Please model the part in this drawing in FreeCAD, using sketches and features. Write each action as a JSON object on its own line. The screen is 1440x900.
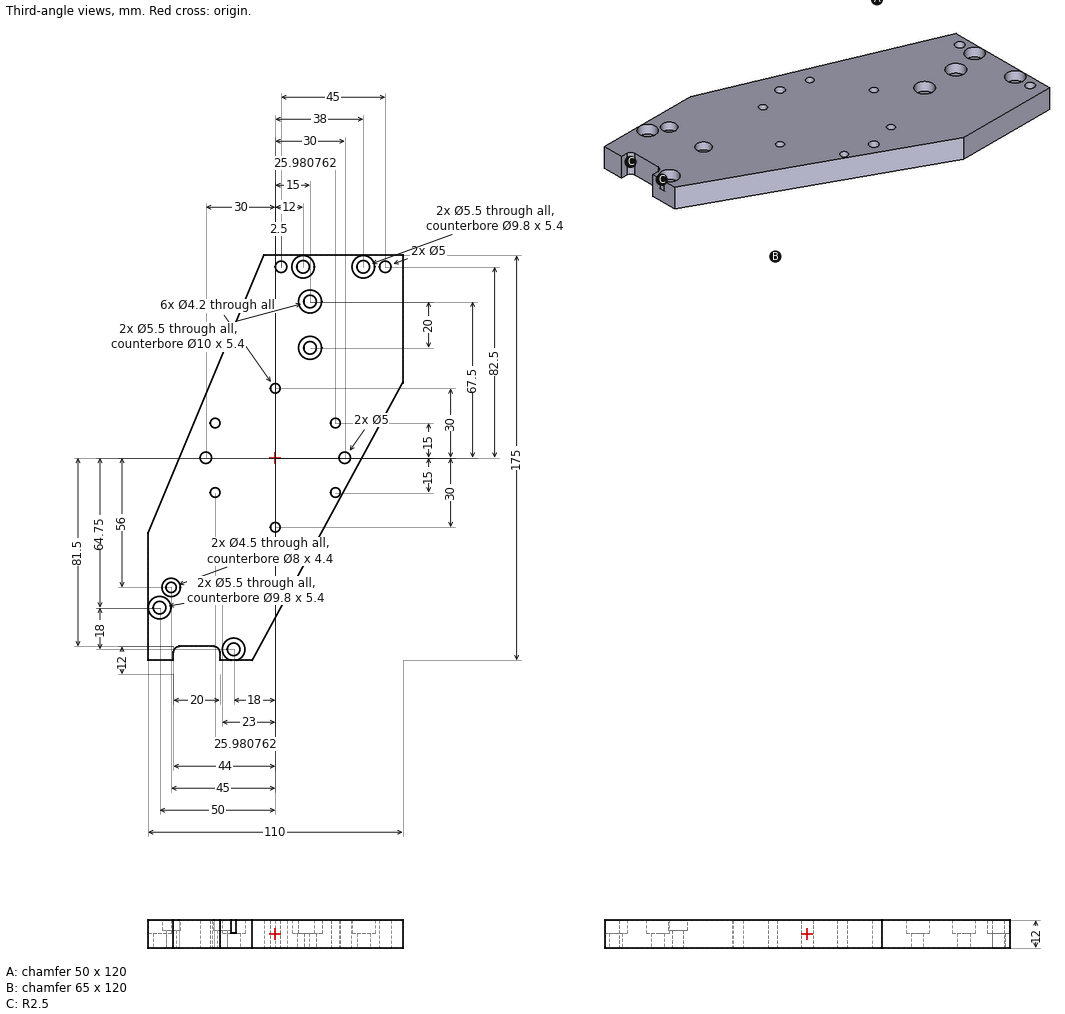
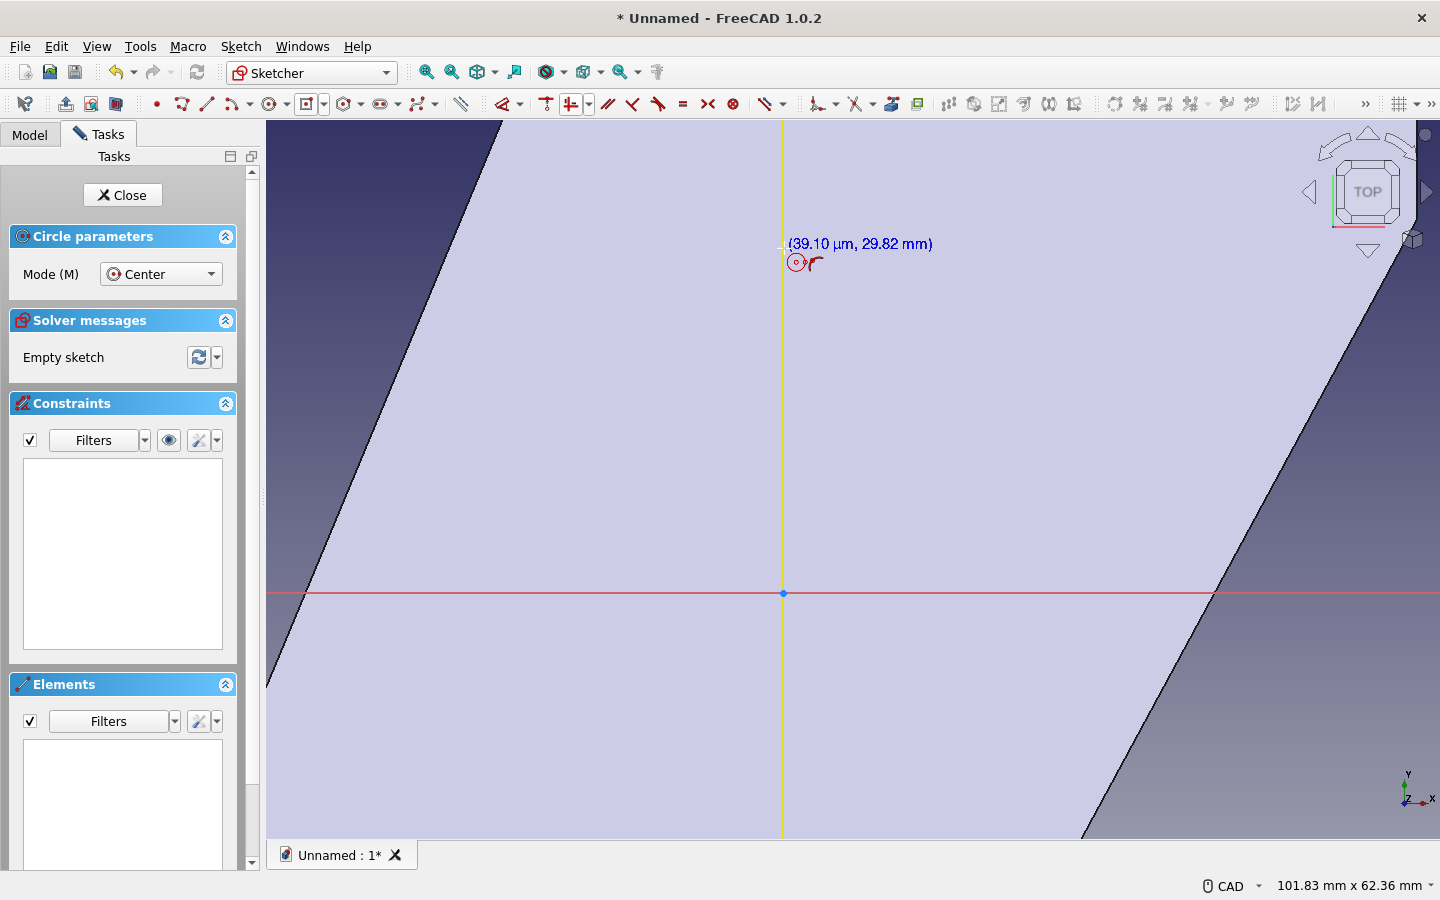
{"action": "left_click", "coordinate": [783, 247]}
{"action": "left_click", "coordinate": [800, 230]}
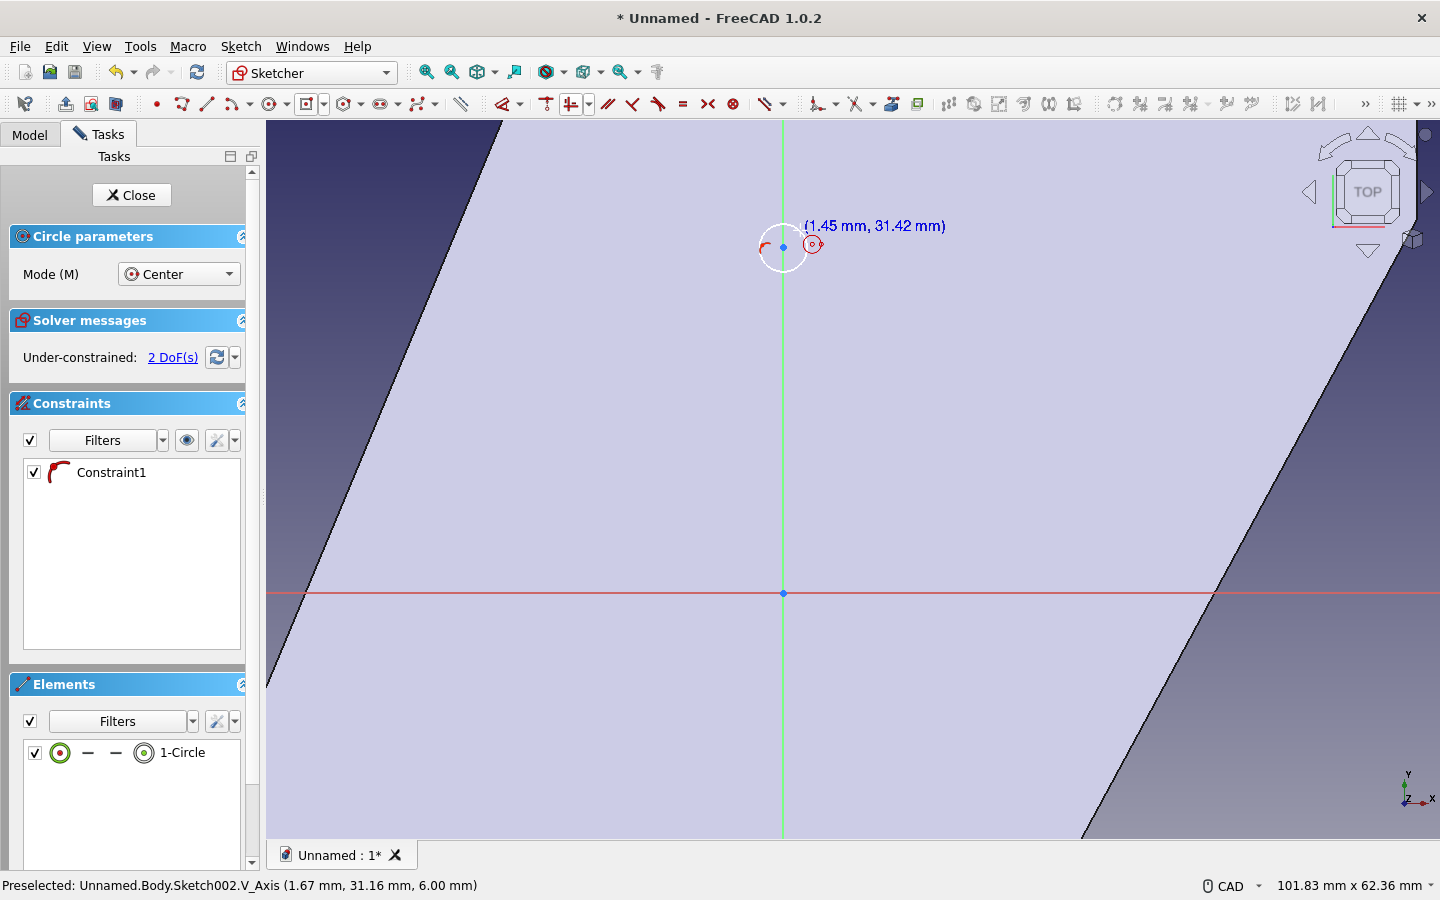
{"action": "left_click", "coordinate": [1083, 420]}
{"action": "left_click", "coordinate": [1100, 403]}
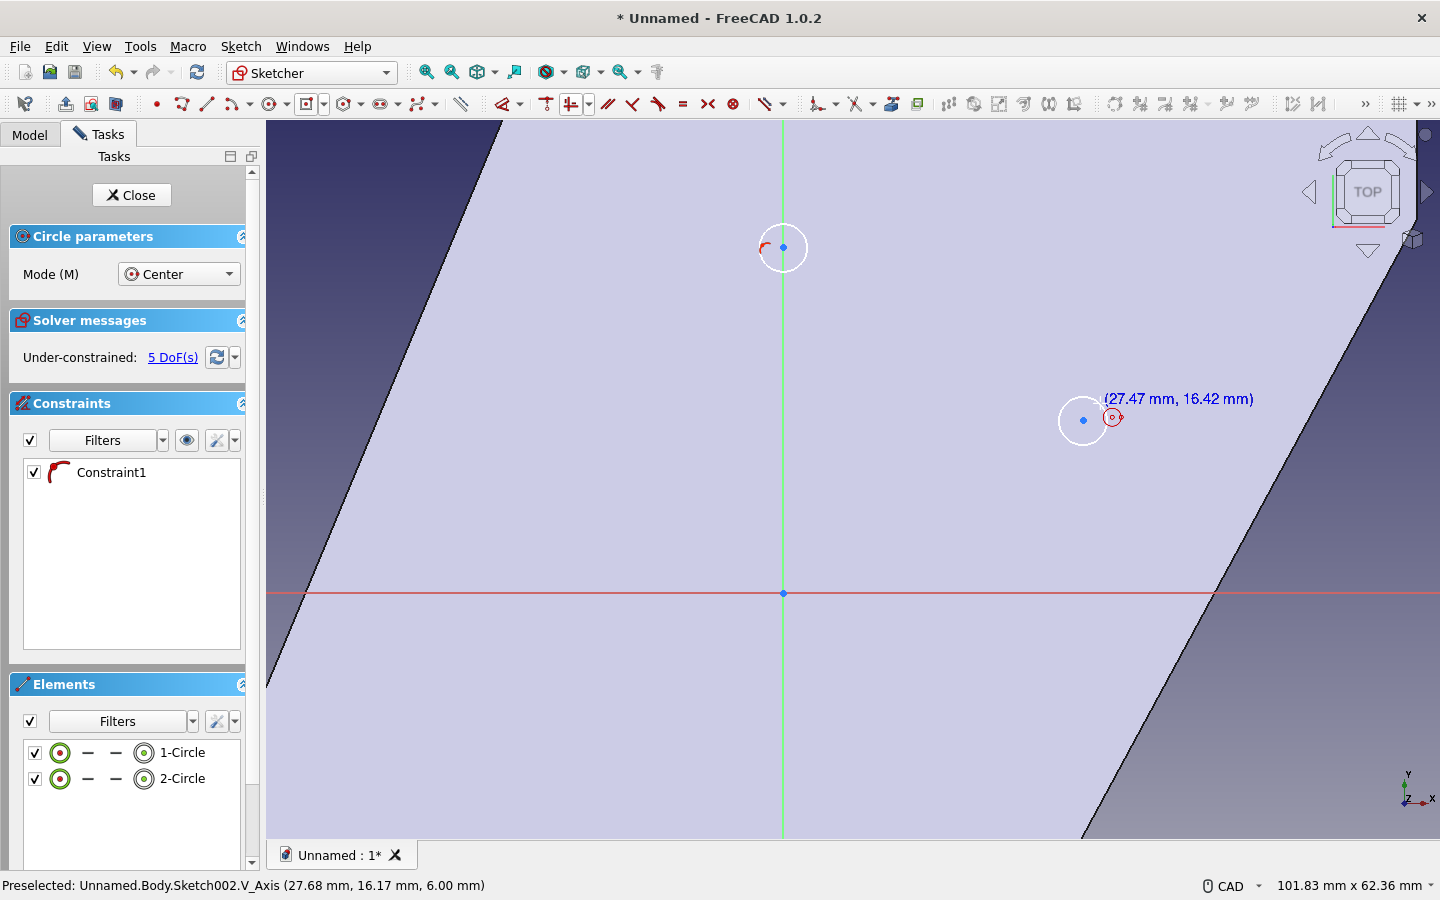
{"action": "left_click", "coordinate": [1083, 766]}
{"action": "left_click", "coordinate": [1100, 749]}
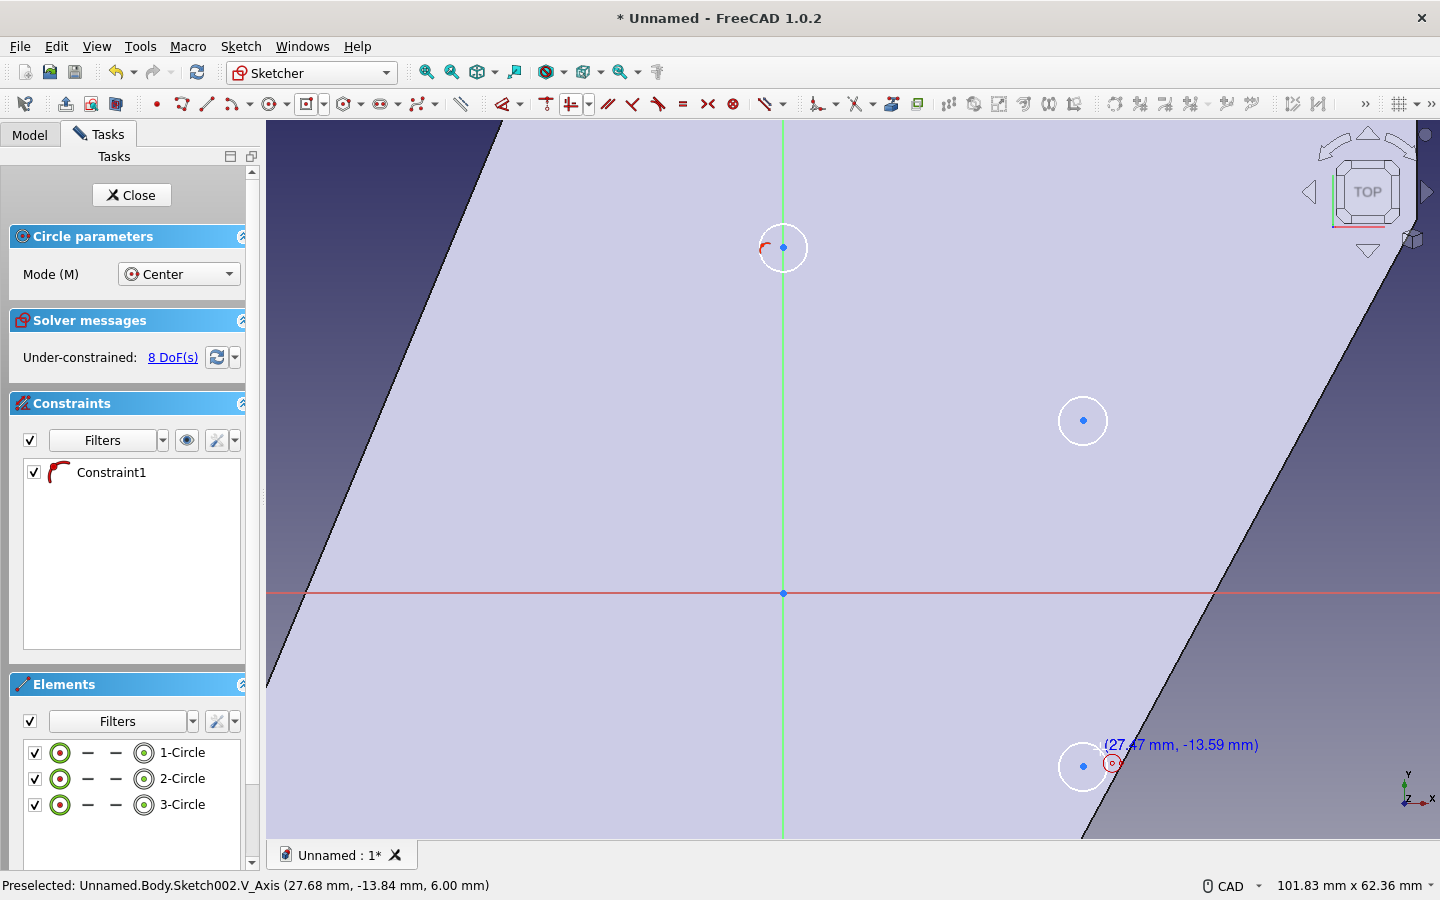
{"action": "scroll", "coordinate": [787, 248], "scroll_direction": "down", "scroll_amount": 2}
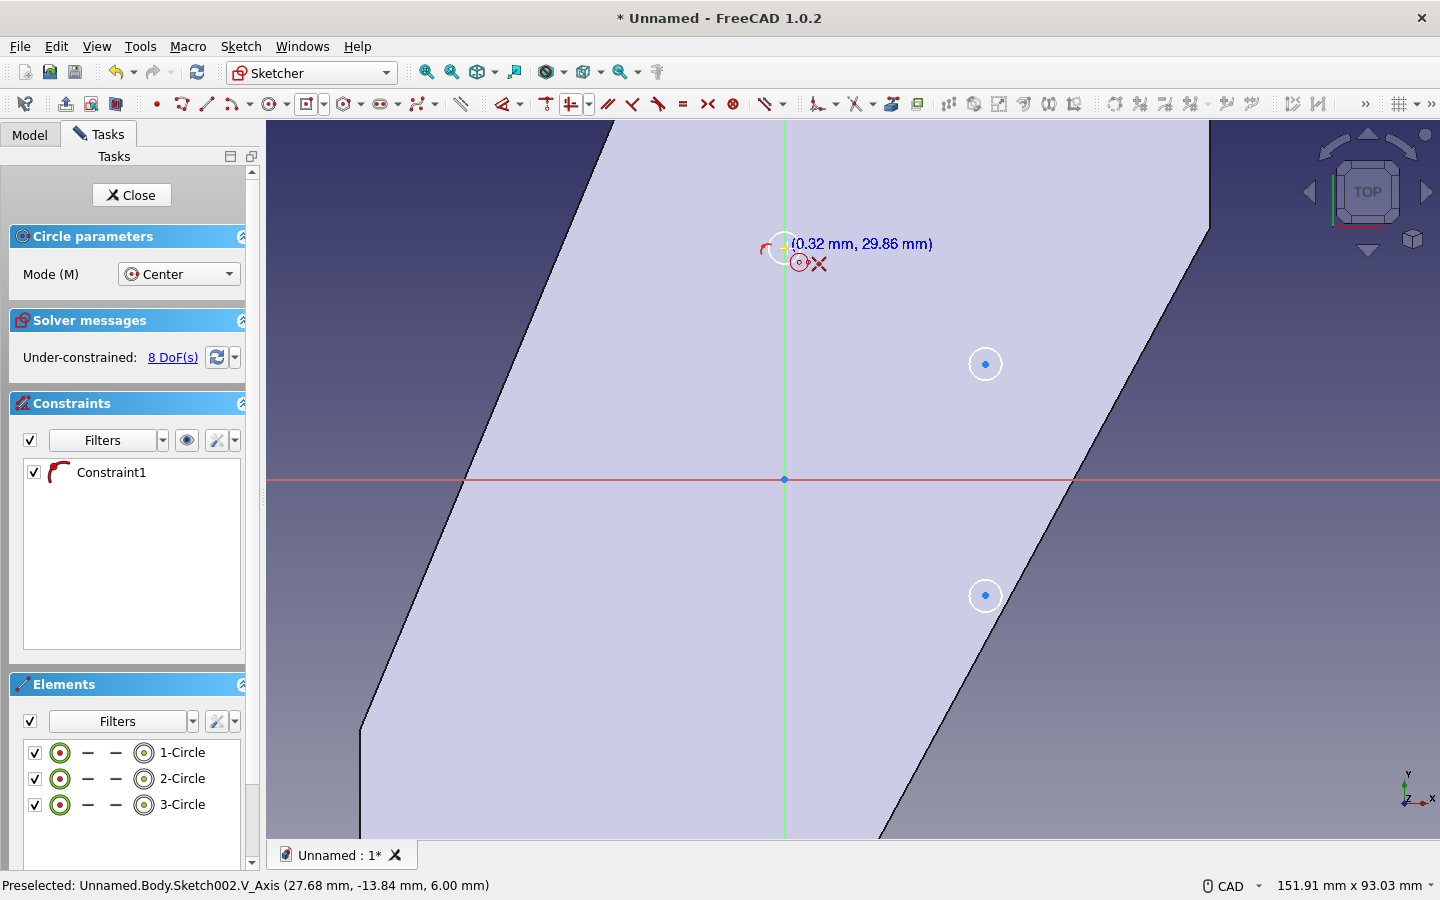
{"action": "scroll", "coordinate": [785, 711], "scroll_direction": "up", "scroll_amount": 2}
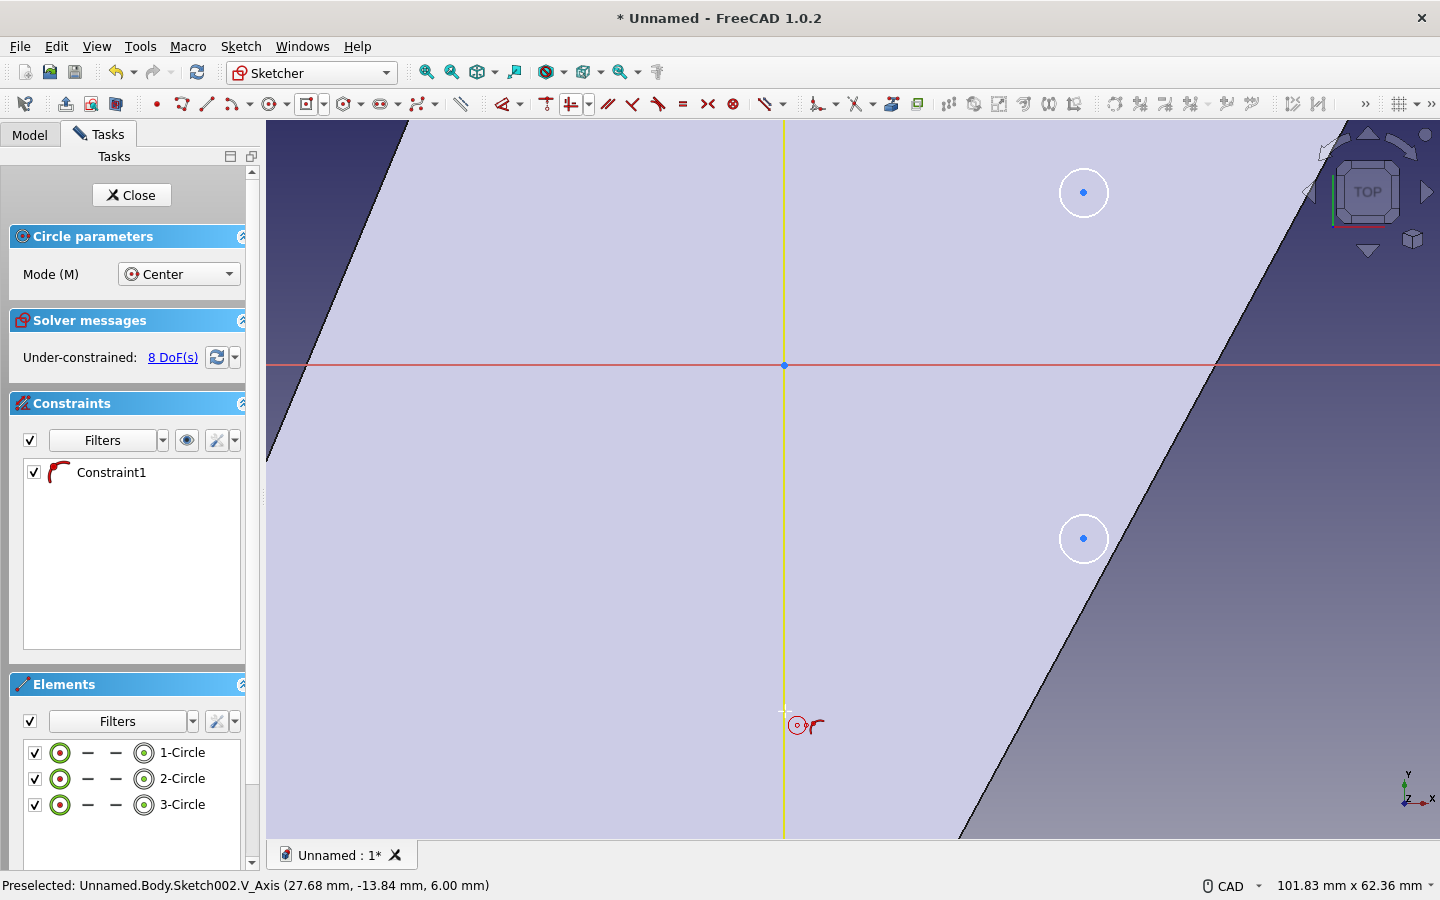
{"action": "left_click", "coordinate": [784, 711]}
{"action": "left_click", "coordinate": [801, 694]}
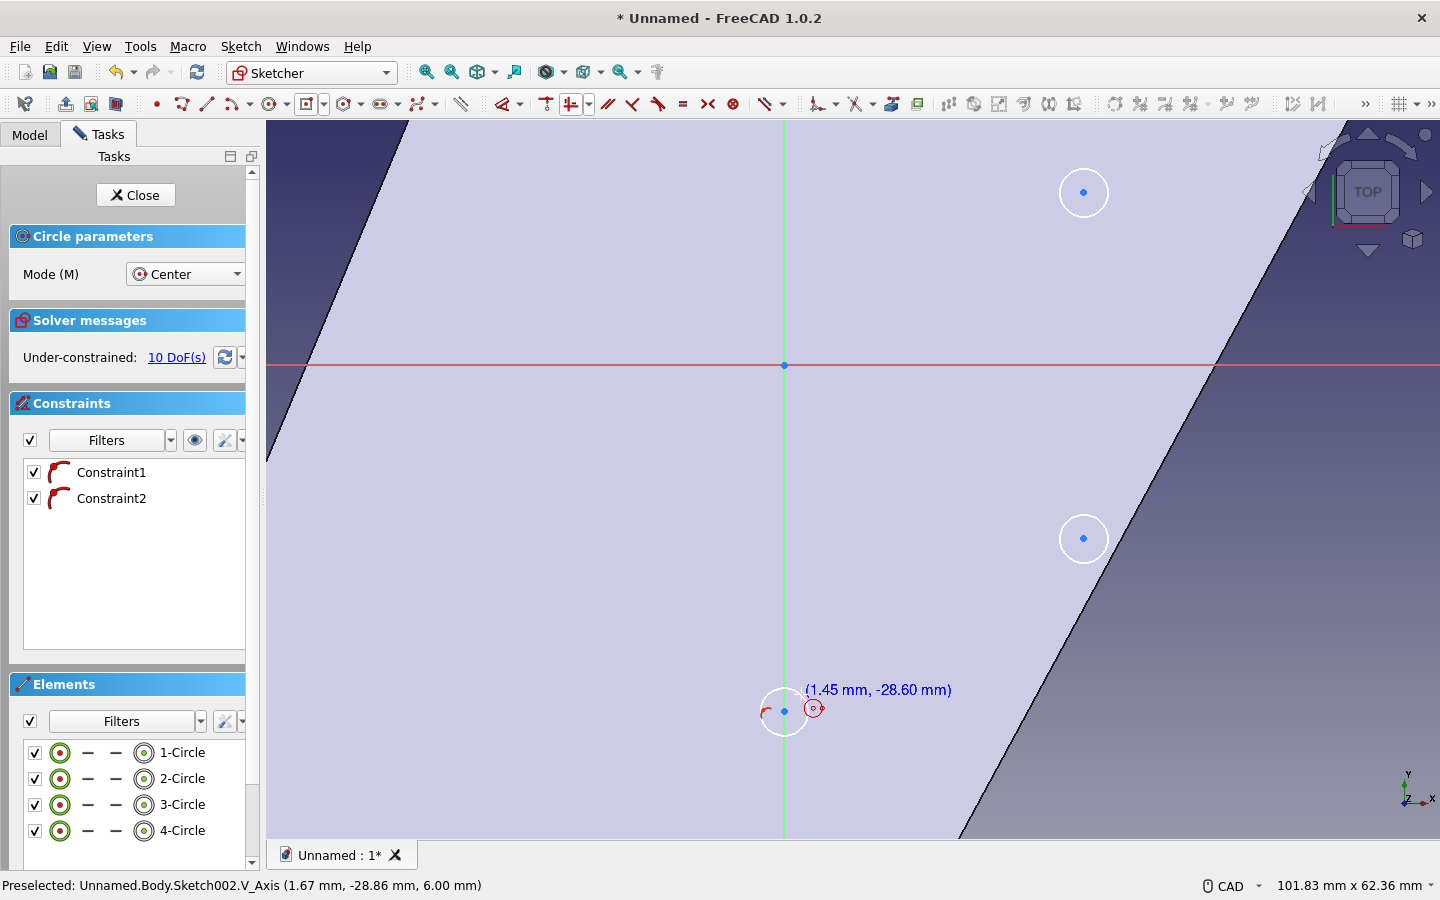
{"action": "left_click", "coordinate": [485, 538]}
{"action": "left_click", "coordinate": [502, 521]}